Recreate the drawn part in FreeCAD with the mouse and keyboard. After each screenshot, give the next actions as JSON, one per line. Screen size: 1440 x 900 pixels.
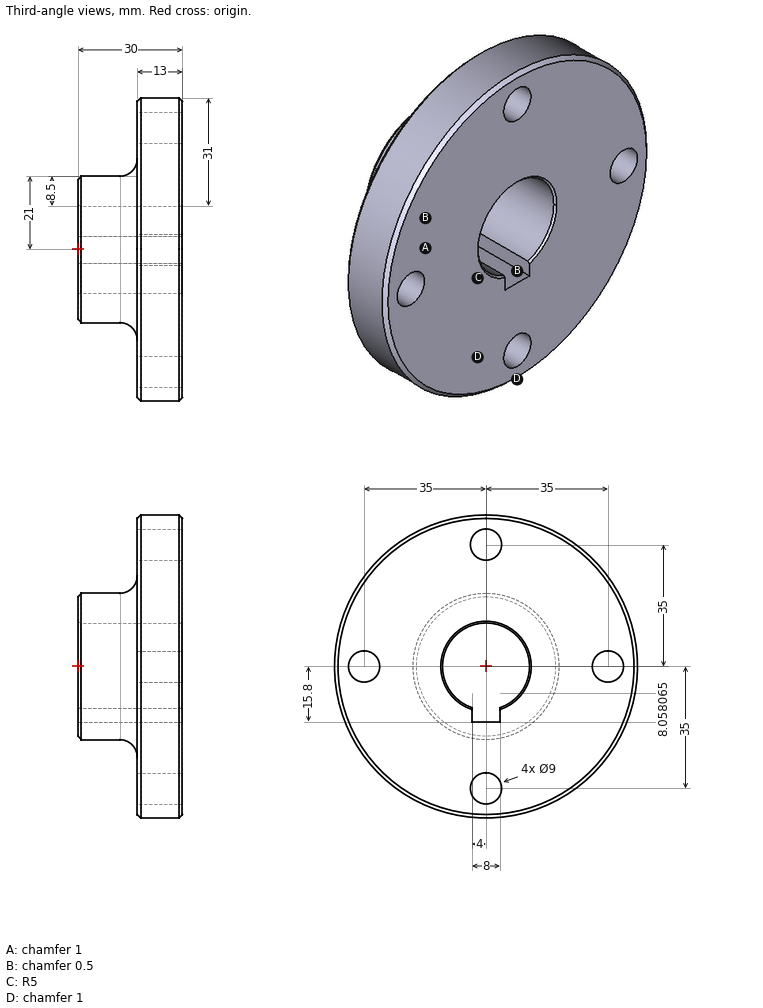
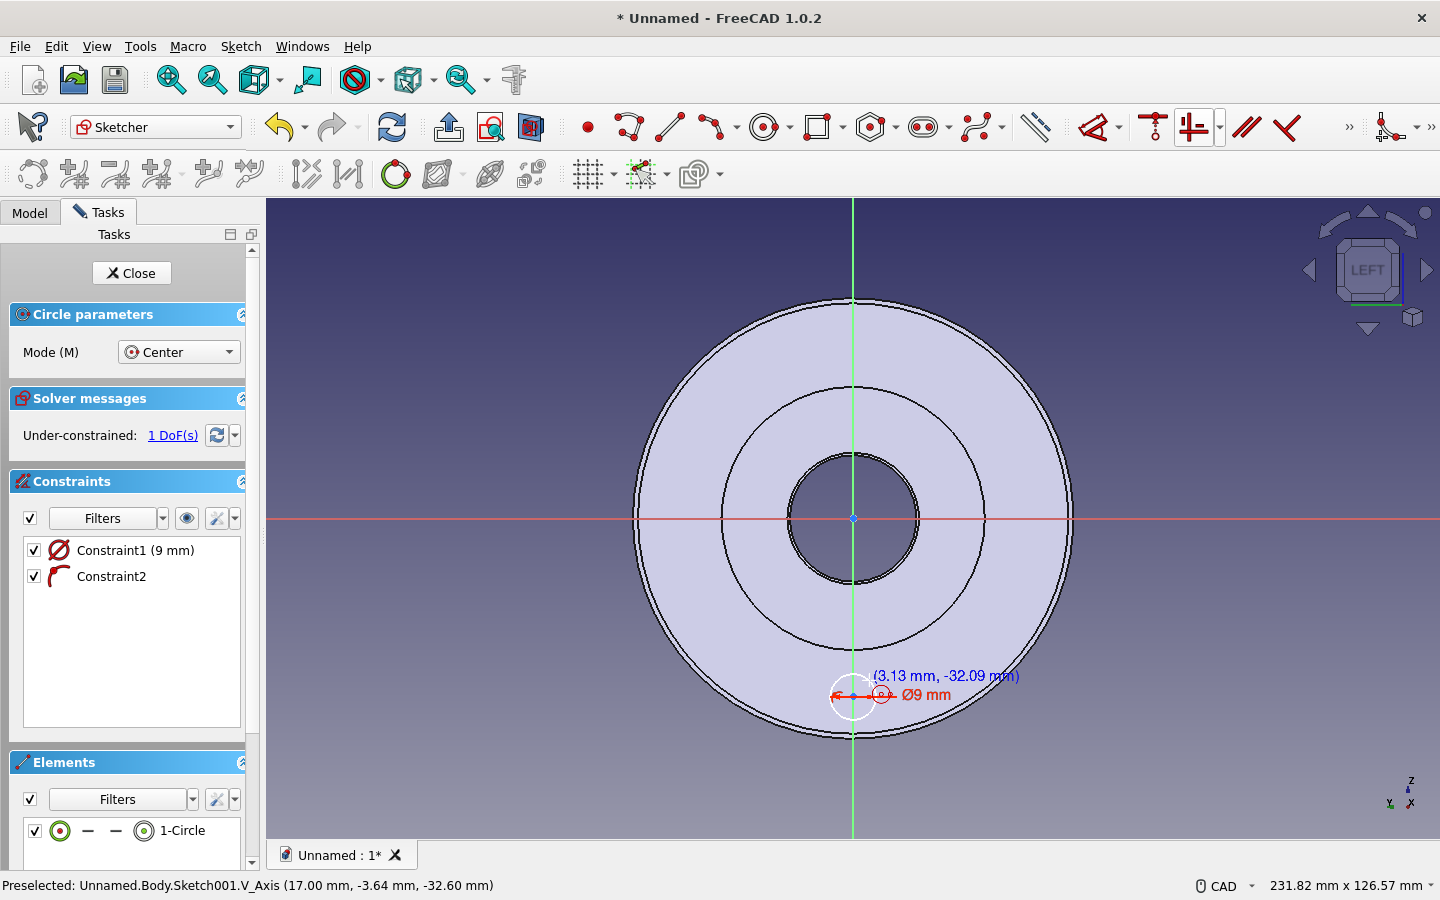
{"action": "left_click", "coordinate": [1030, 518]}
{"action": "mouse_move", "coordinate": [1047, 502]}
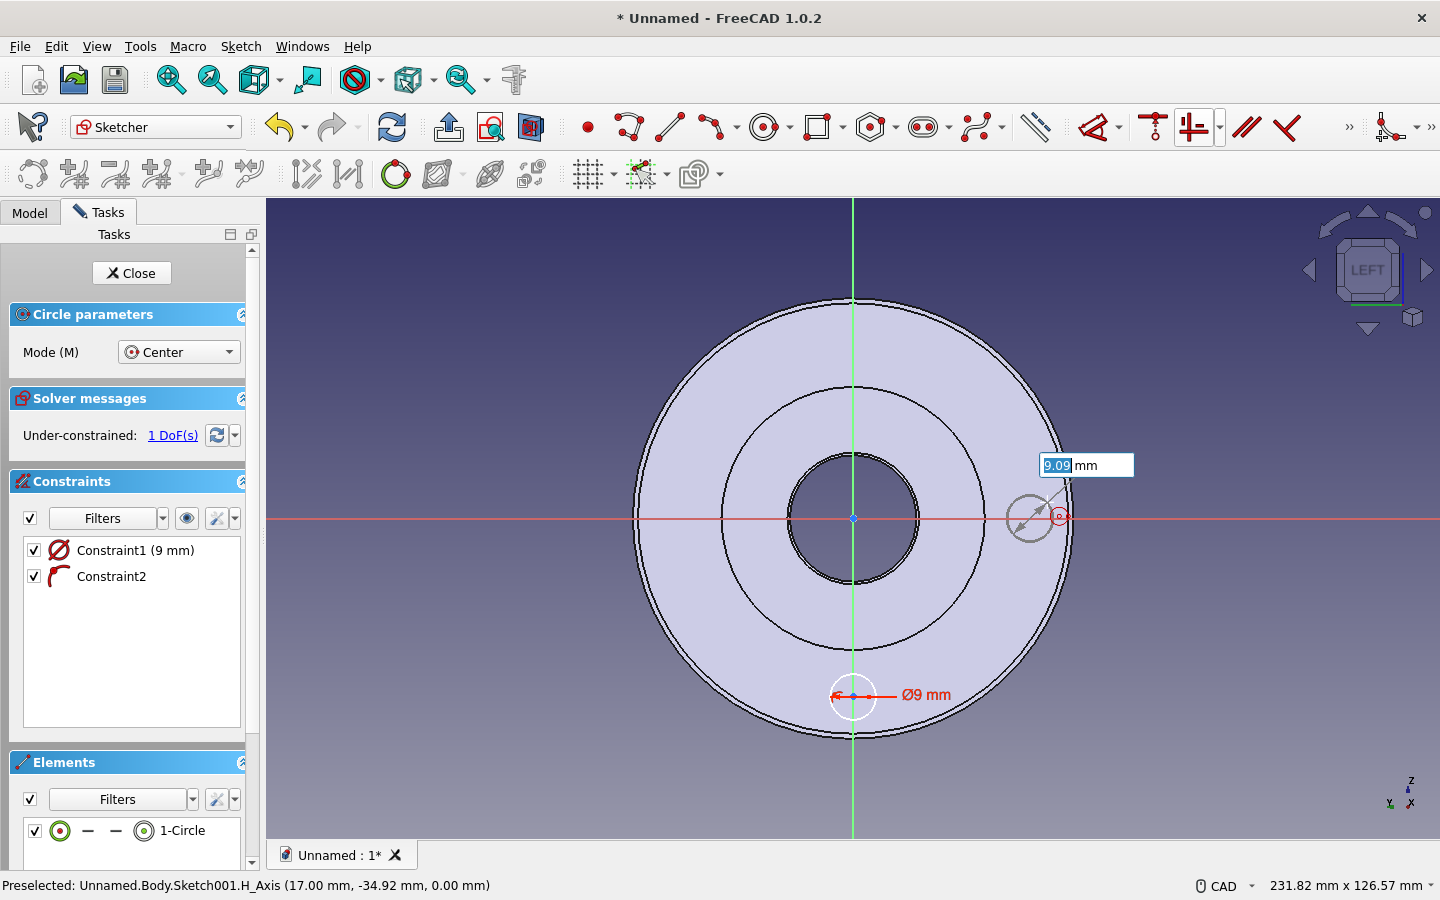
{"action": "type", "text": "9"}
{"action": "key", "text": "Return"}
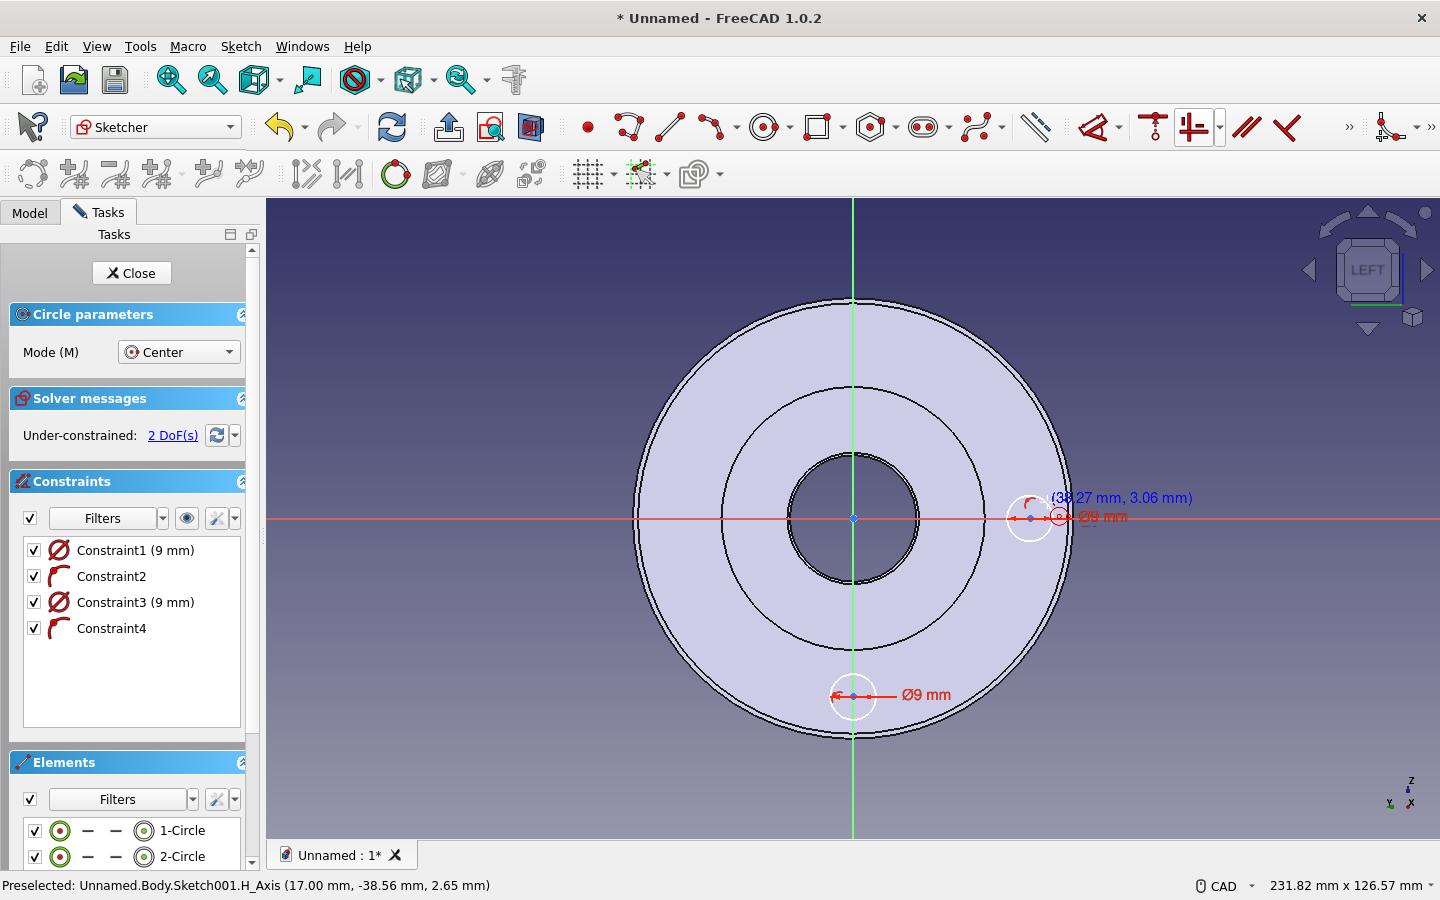
{"action": "left_click", "coordinate": [676, 518]}
{"action": "mouse_move", "coordinate": [692, 502]}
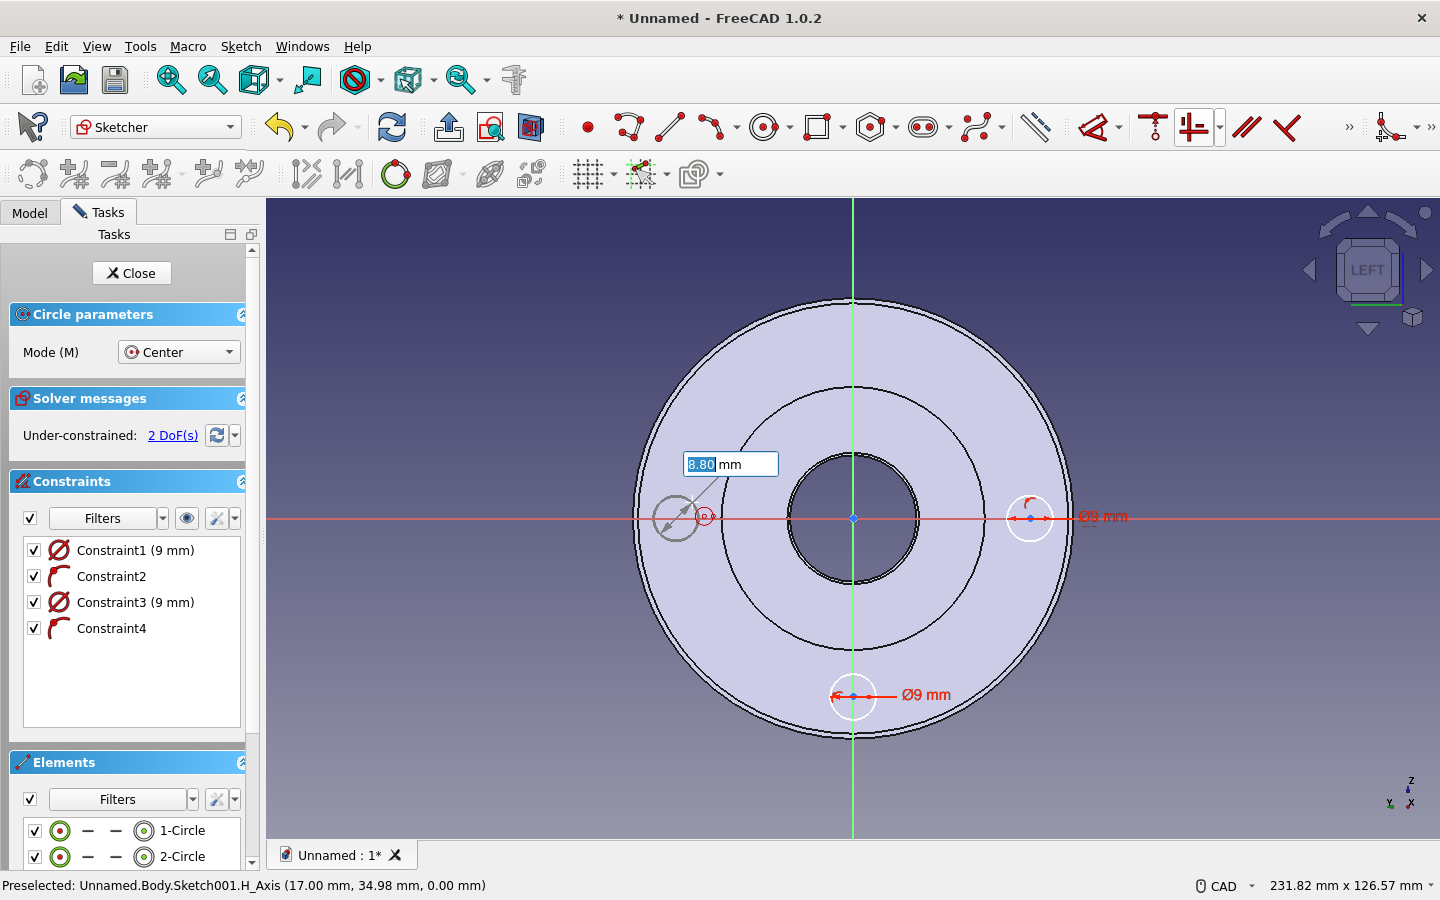
{"action": "type", "text": "9"}
{"action": "key", "text": "Return"}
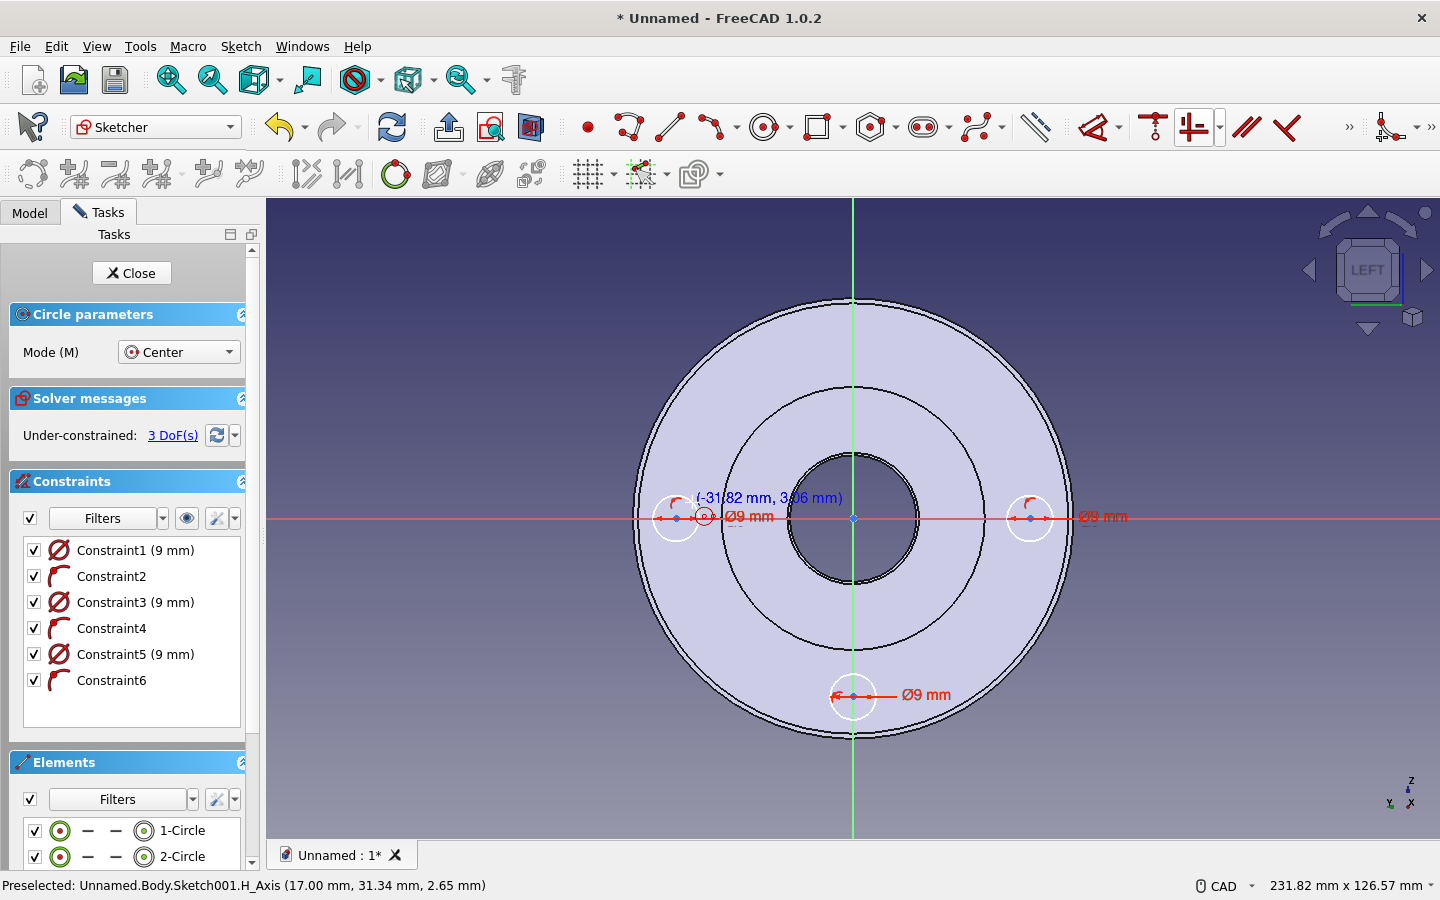
{"action": "left_click", "coordinate": [853, 341]}
{"action": "mouse_move", "coordinate": [869, 325]}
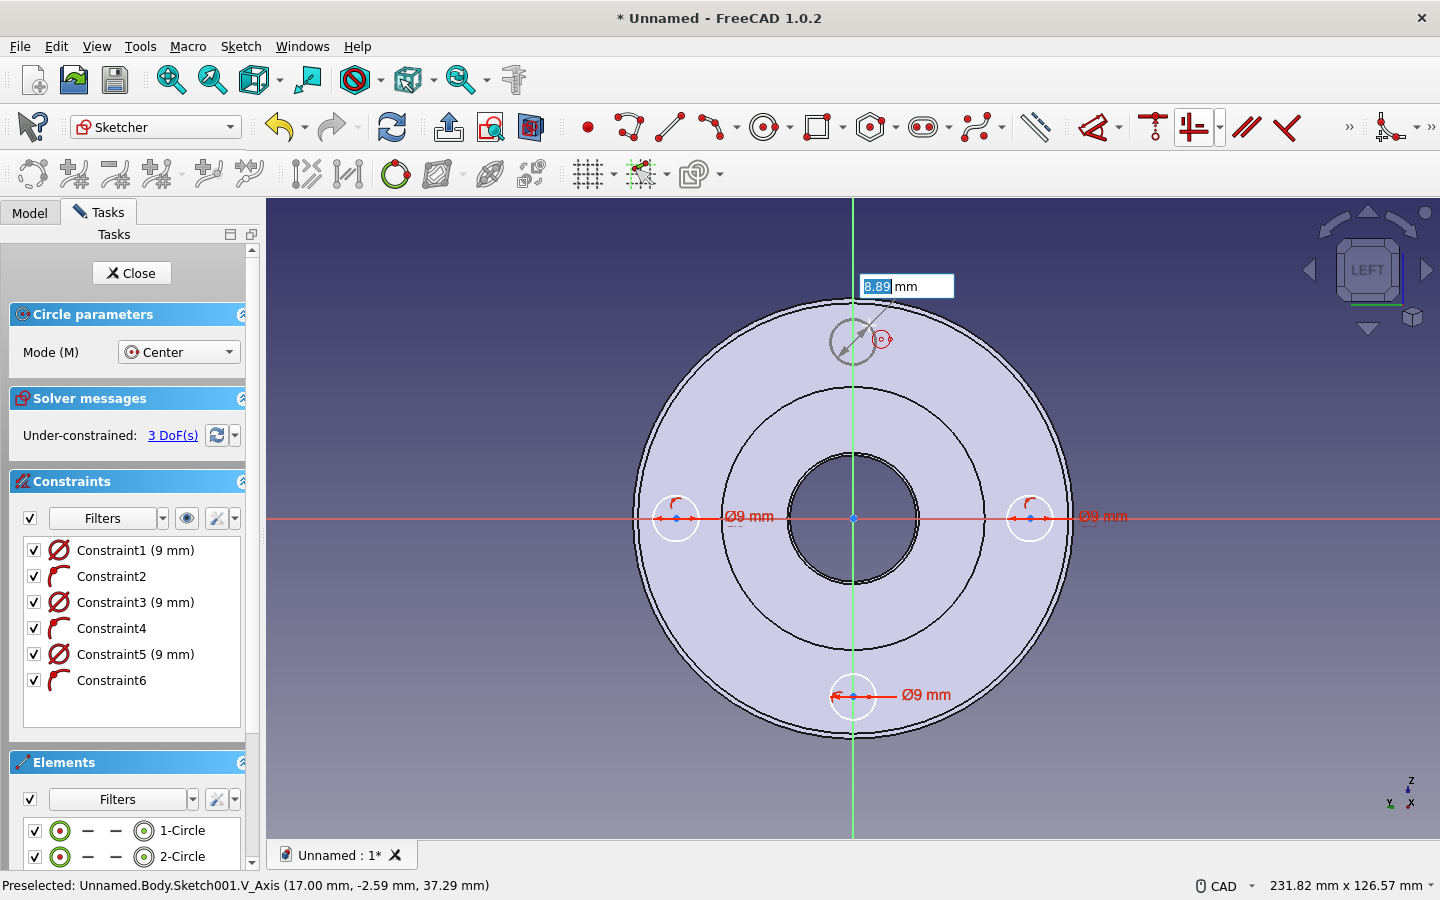
{"action": "type", "text": "9"}
{"action": "key", "text": "Return"}
{"action": "key", "text": "Escape"}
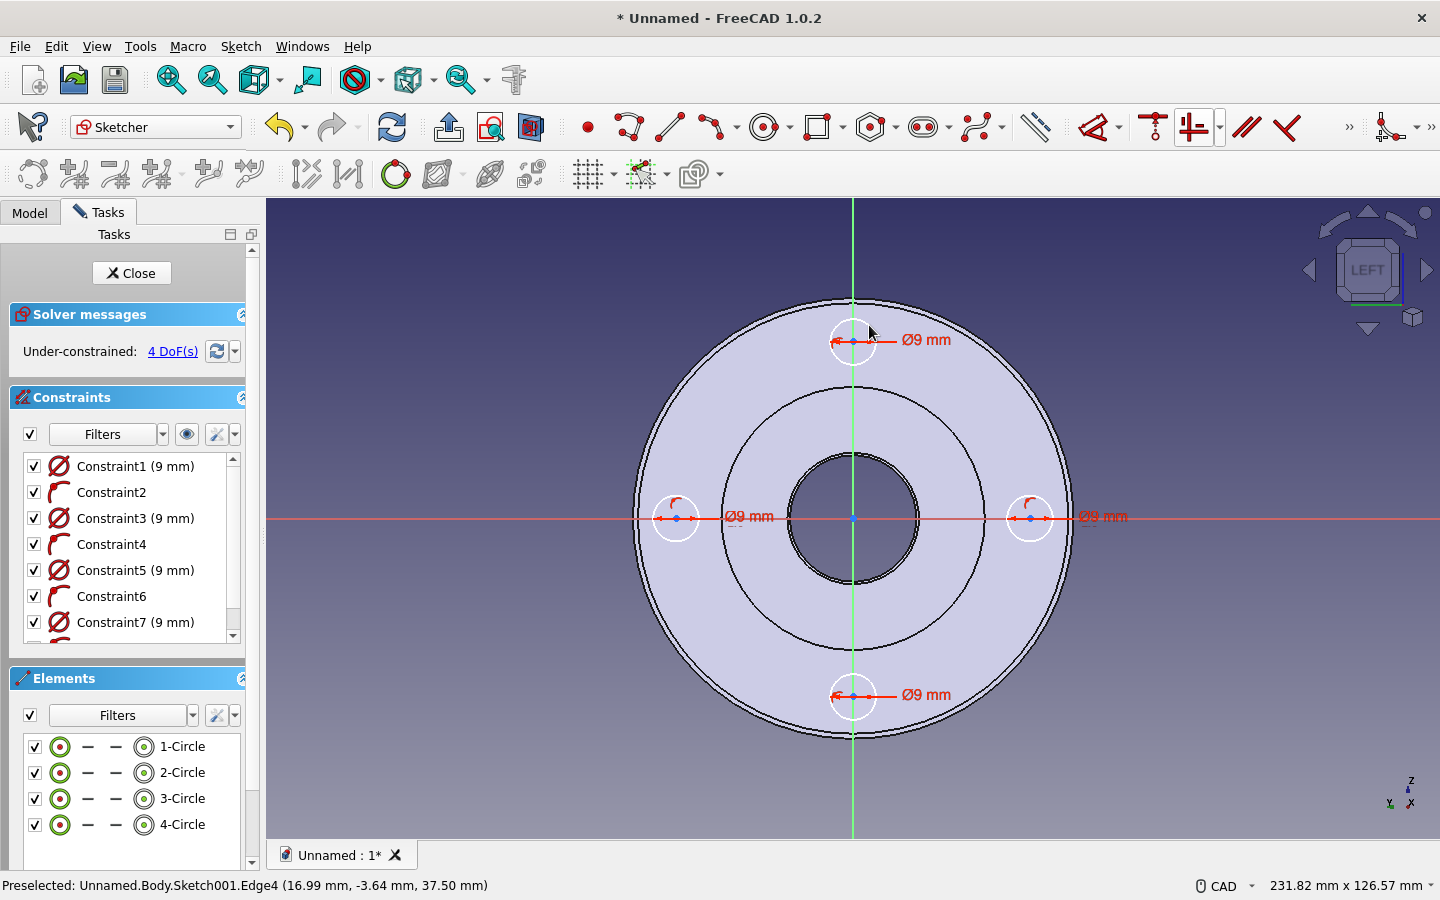
{"action": "left_click", "coordinate": [1092, 128]}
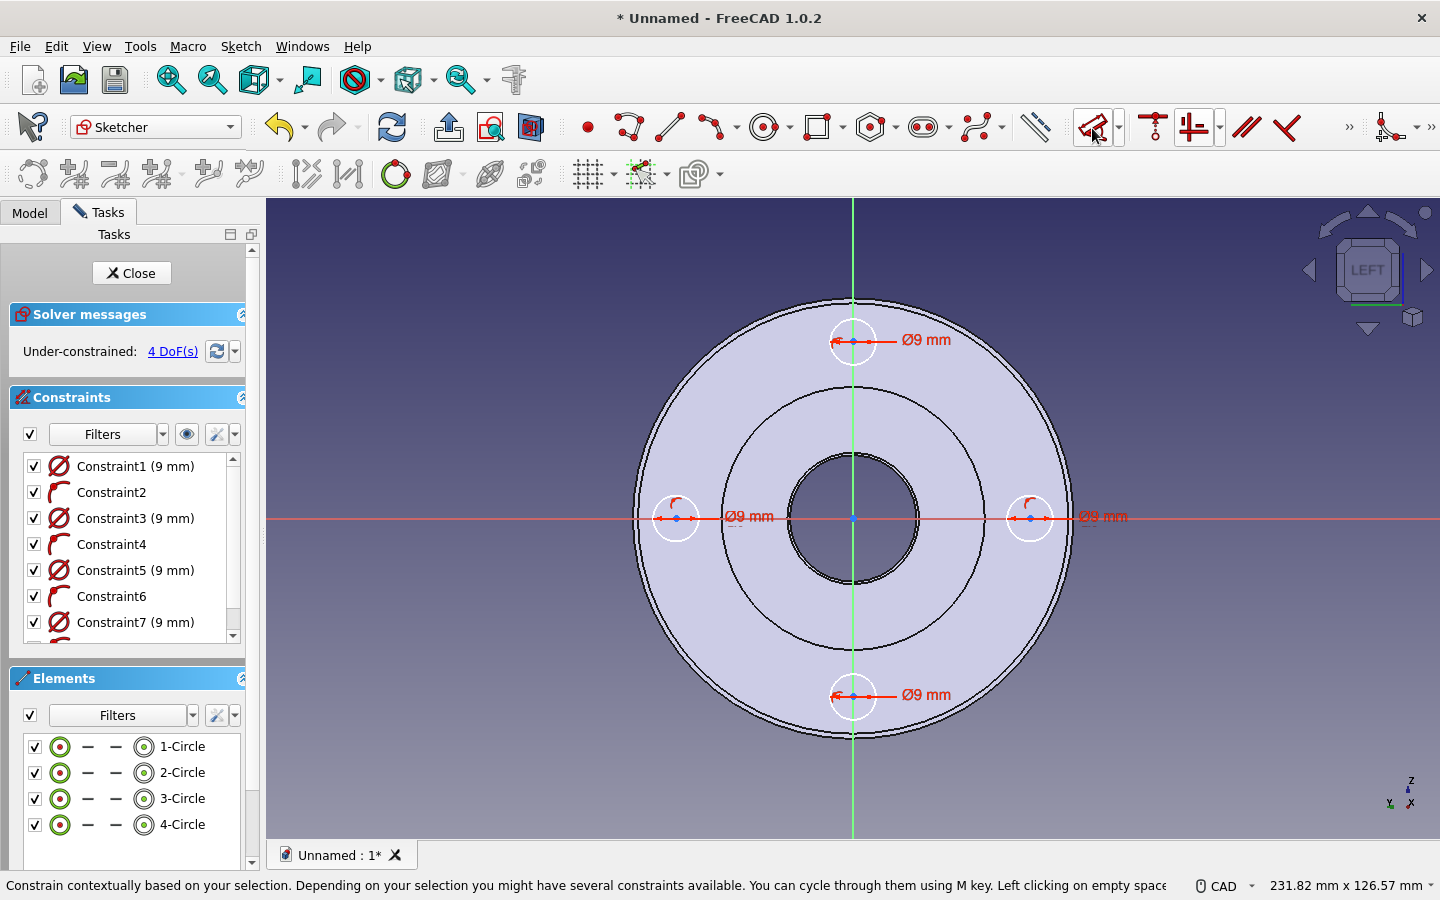
{"action": "left_click", "coordinate": [853, 697]}
{"action": "left_click", "coordinate": [887, 608]}